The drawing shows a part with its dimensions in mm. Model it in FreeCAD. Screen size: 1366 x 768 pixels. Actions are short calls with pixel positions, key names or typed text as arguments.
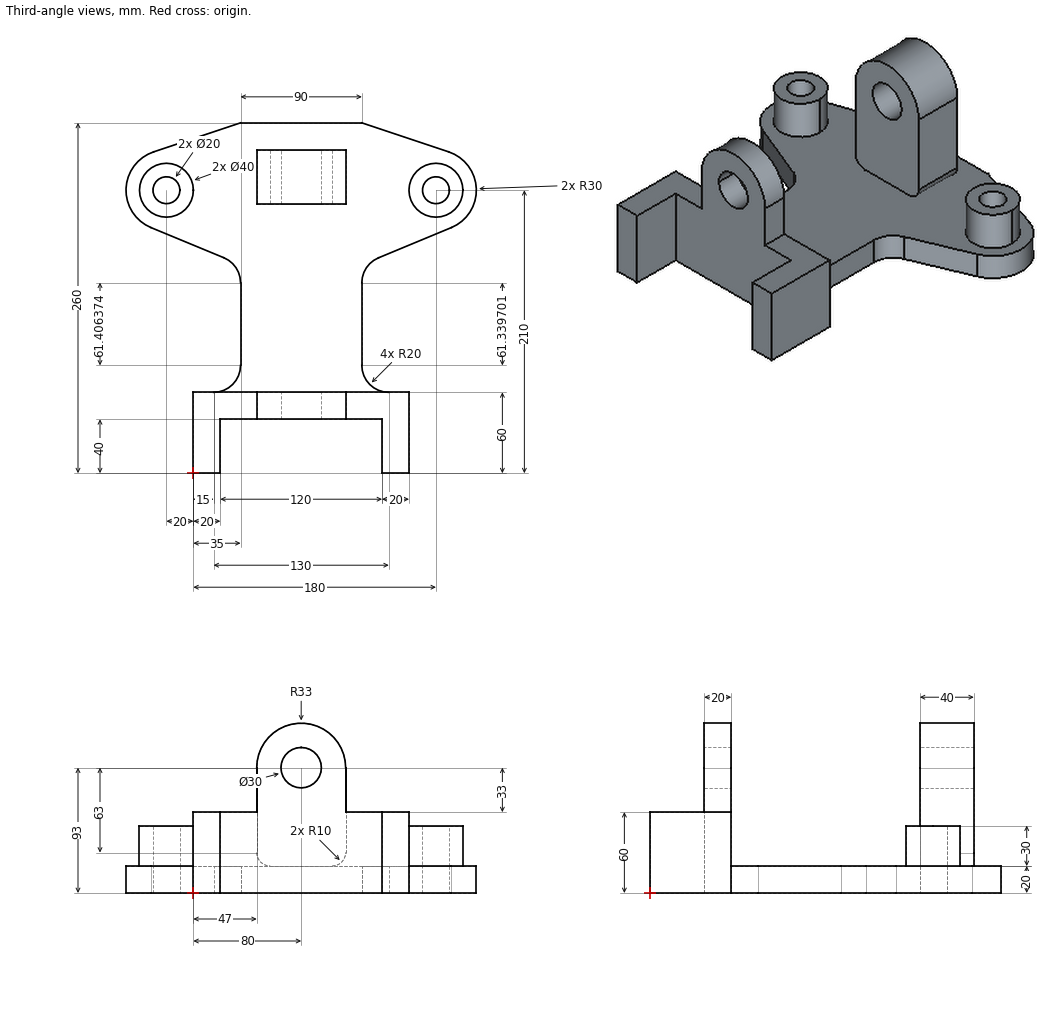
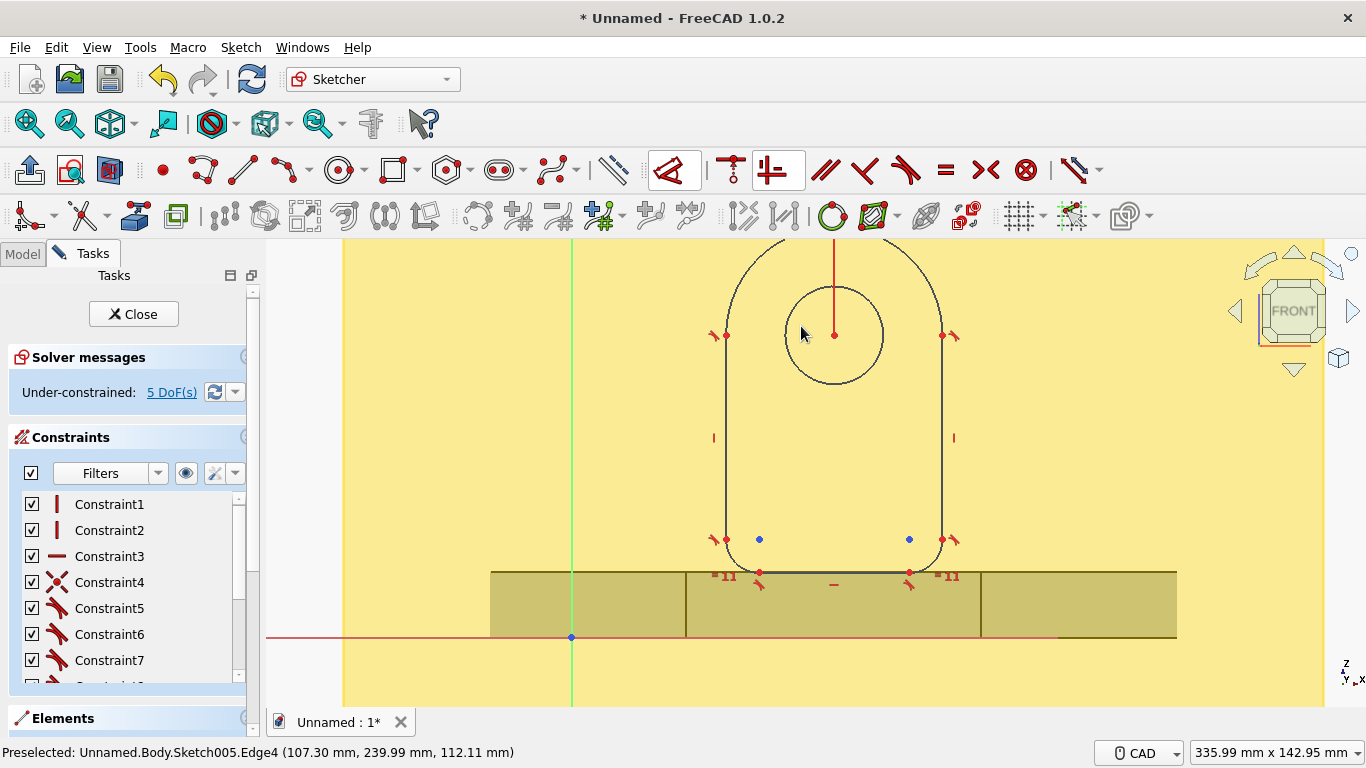
click(924, 569)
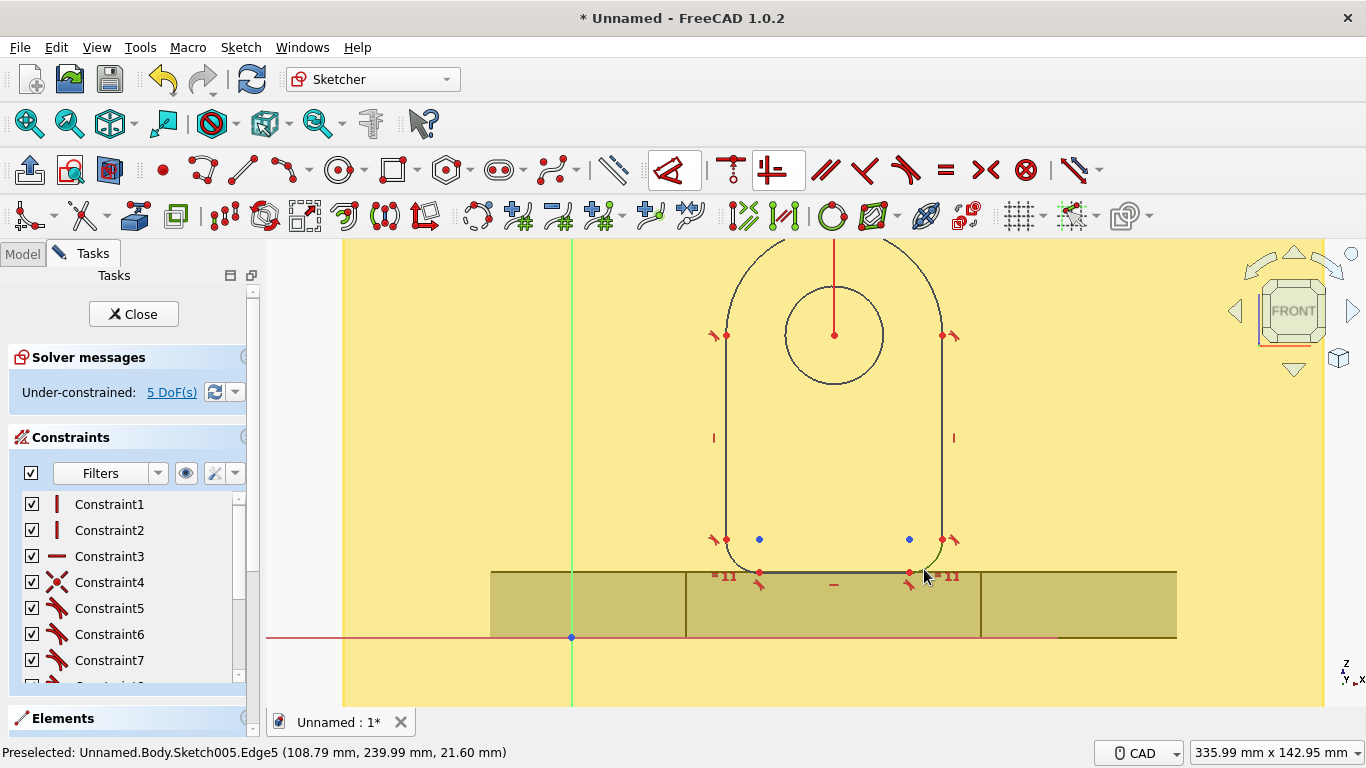
click(696, 170)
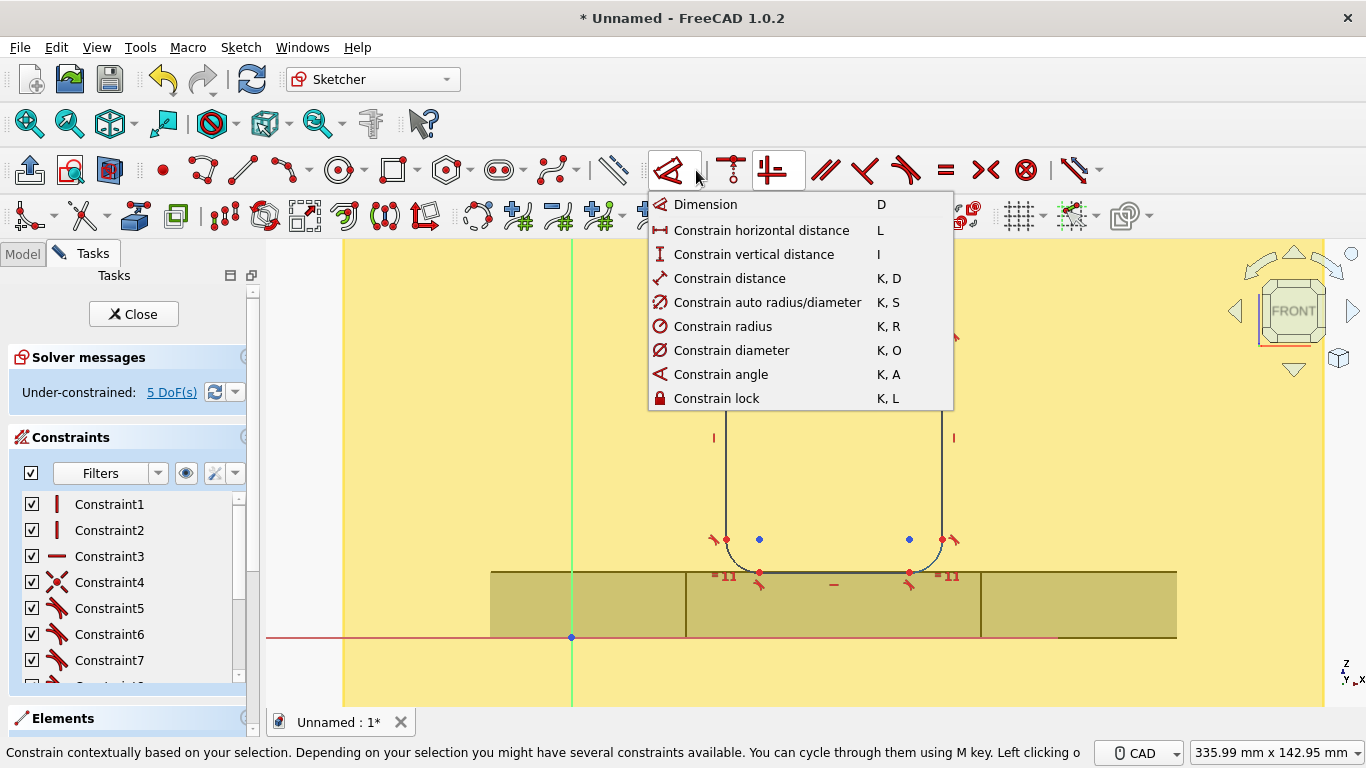
click(801, 326)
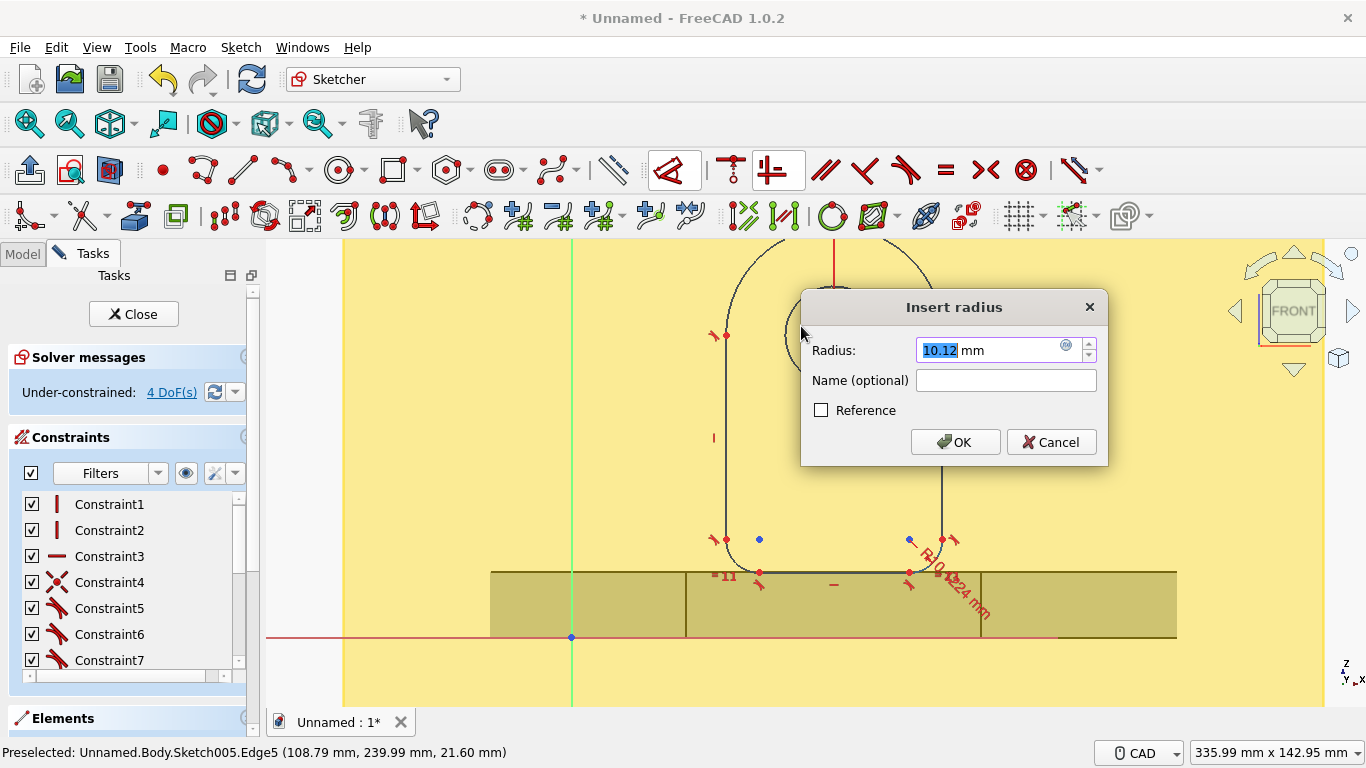
text(10)
key(Return)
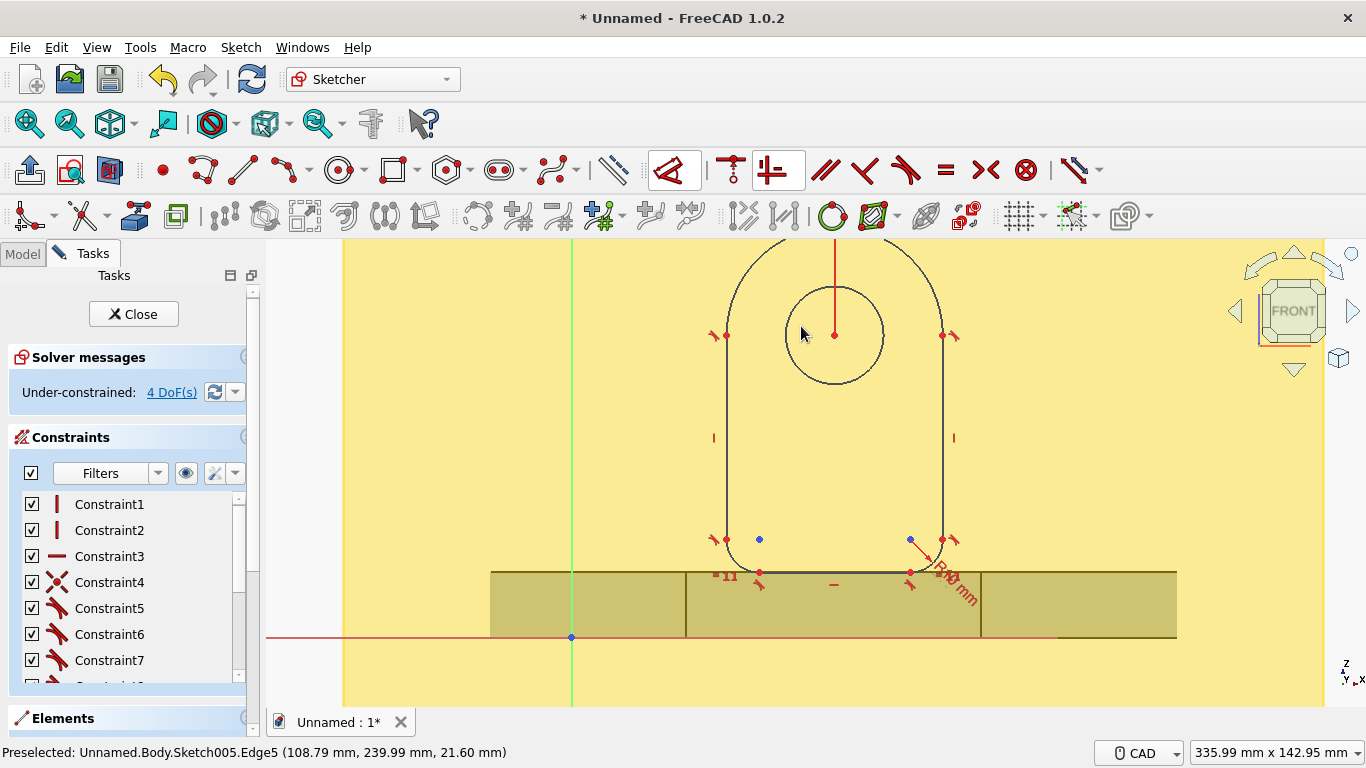
click(869, 301)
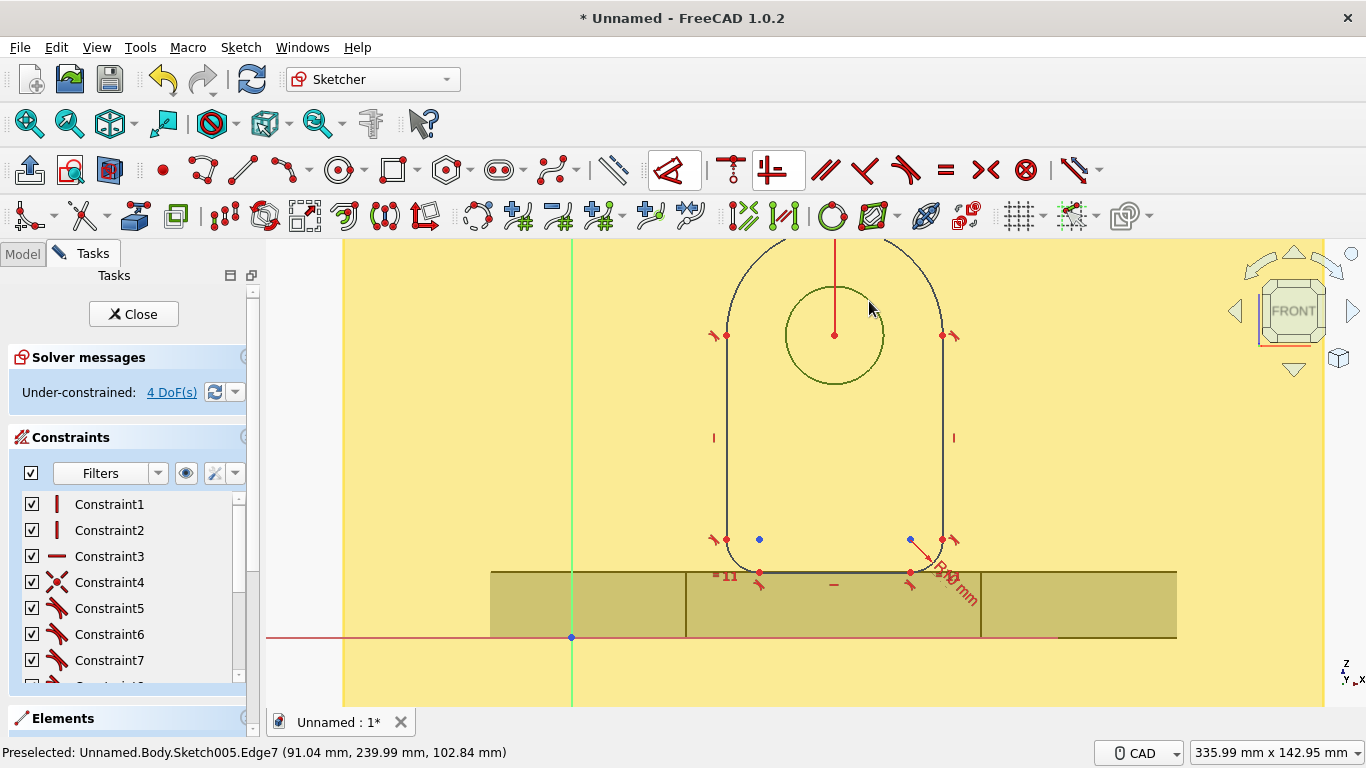
key(k)
key(o)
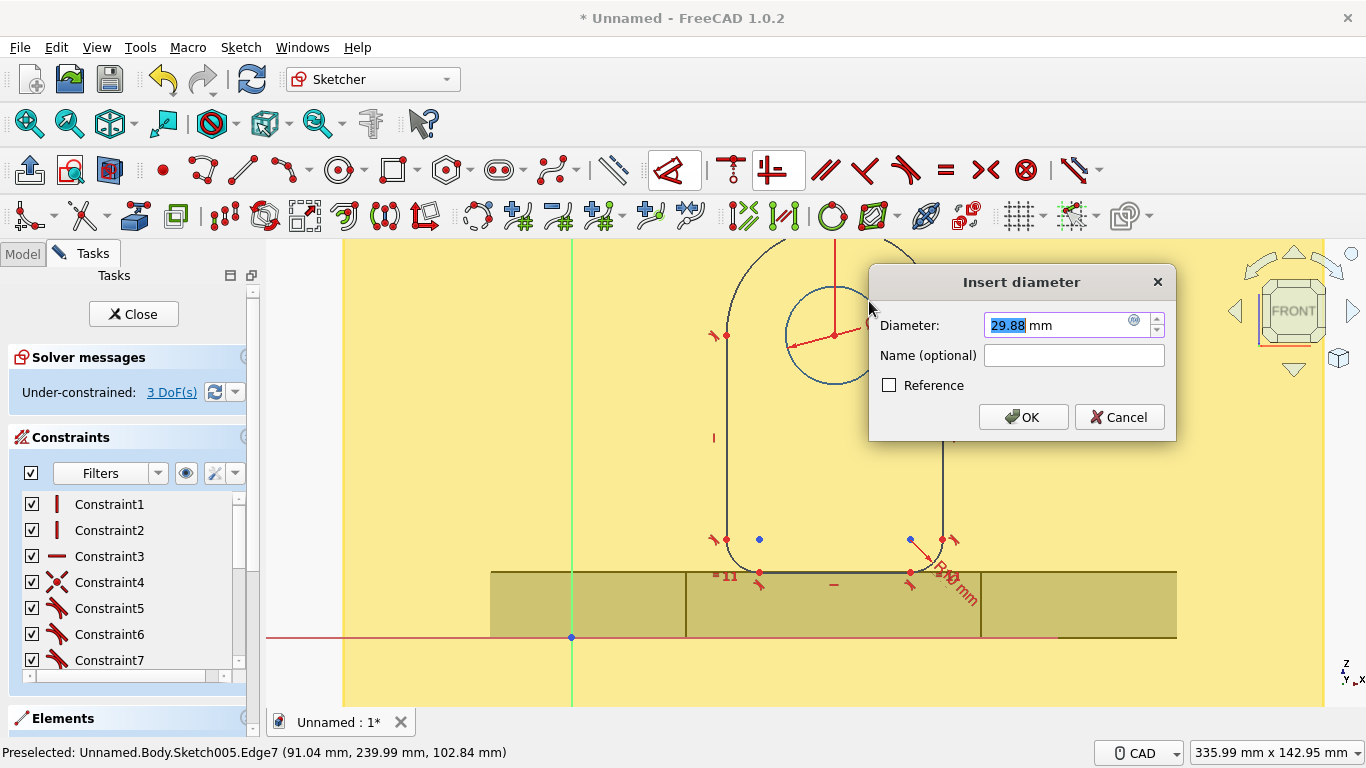
text(30)
key(Return)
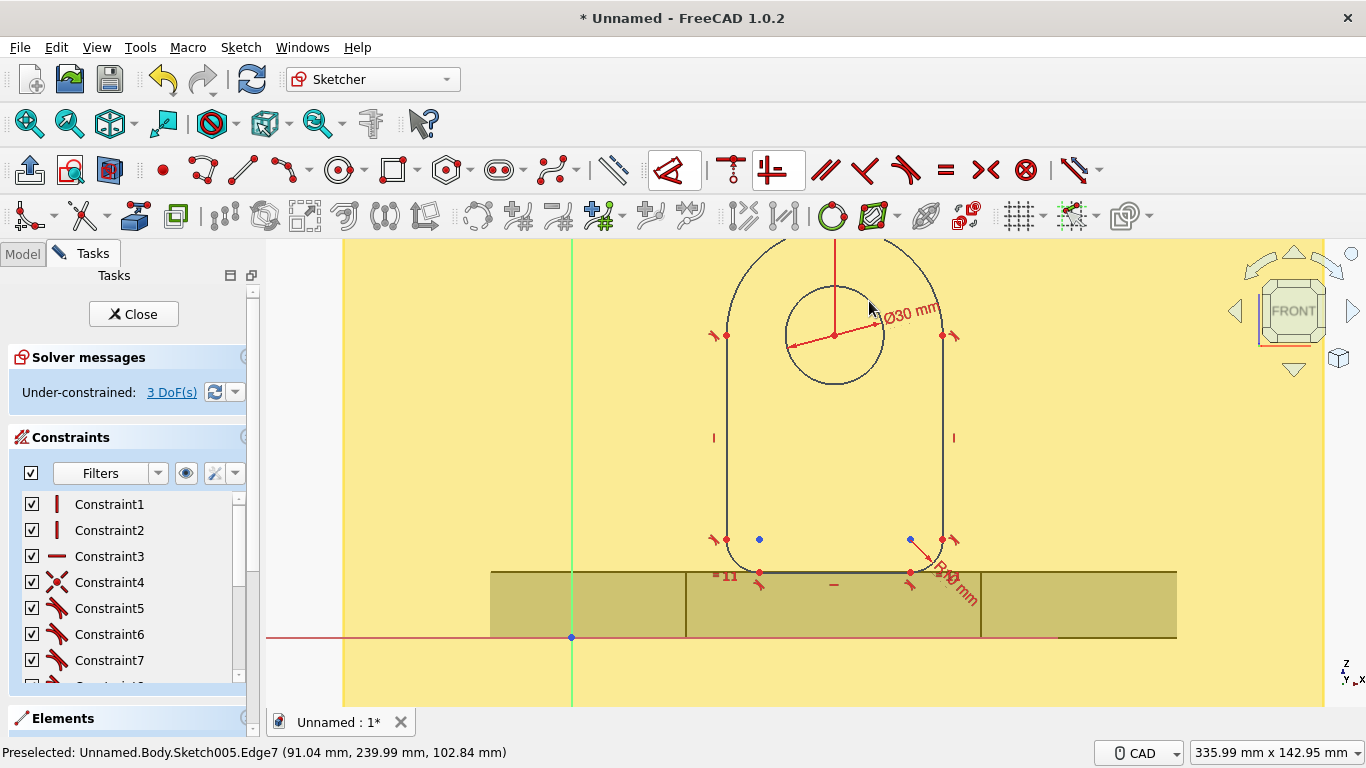
click(727, 478)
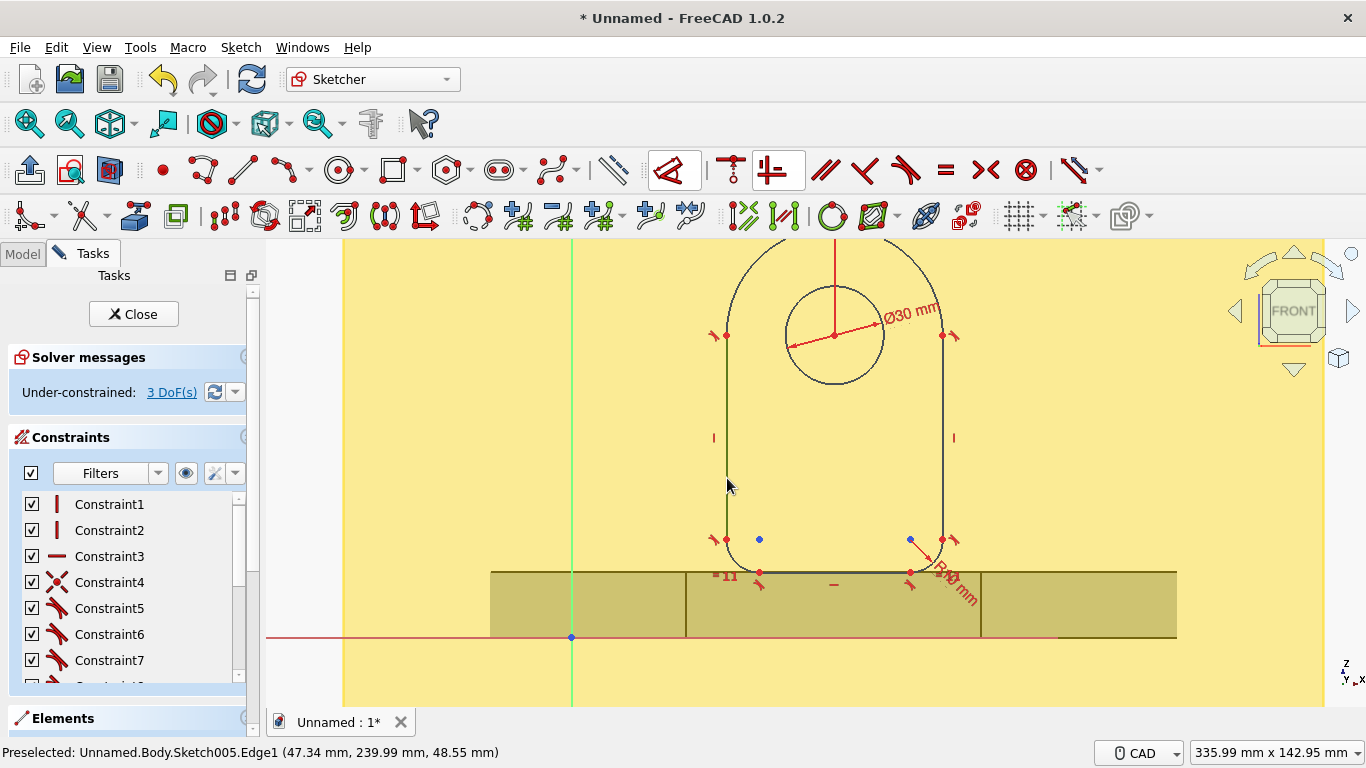
key(i)